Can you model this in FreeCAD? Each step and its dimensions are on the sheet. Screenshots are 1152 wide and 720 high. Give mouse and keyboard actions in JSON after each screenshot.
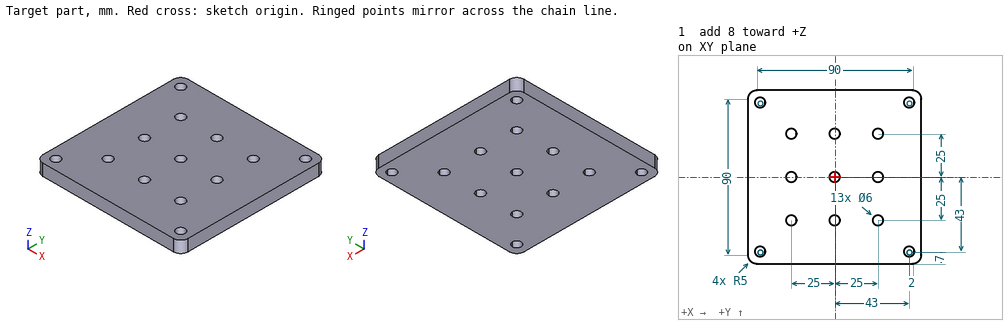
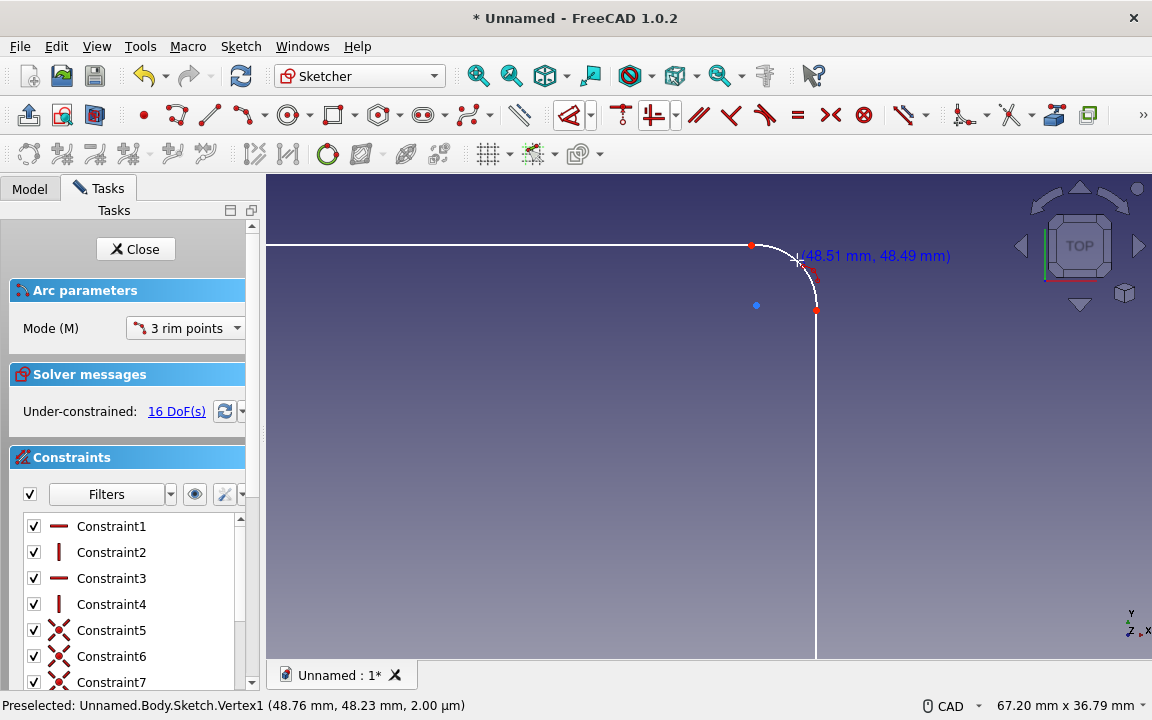
{"action": "left_click", "coordinate": [288, 116]}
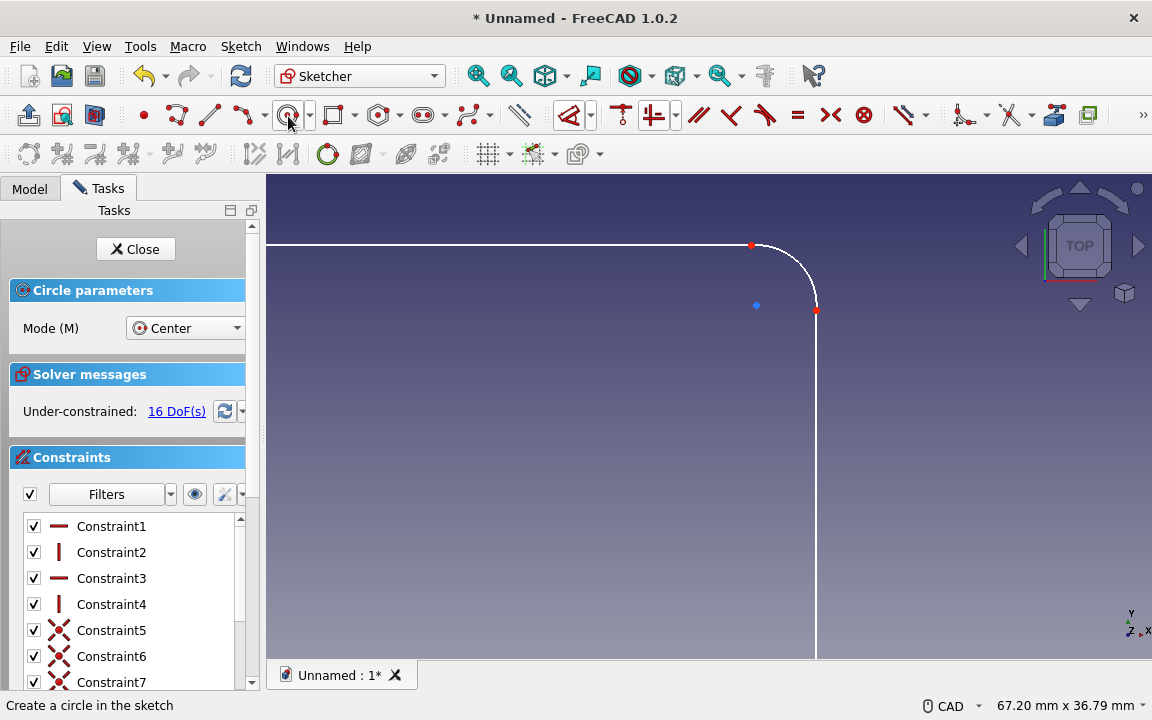
{"action": "scroll", "coordinate": [799, 258], "scroll_direction": "down", "scroll_amount": 7}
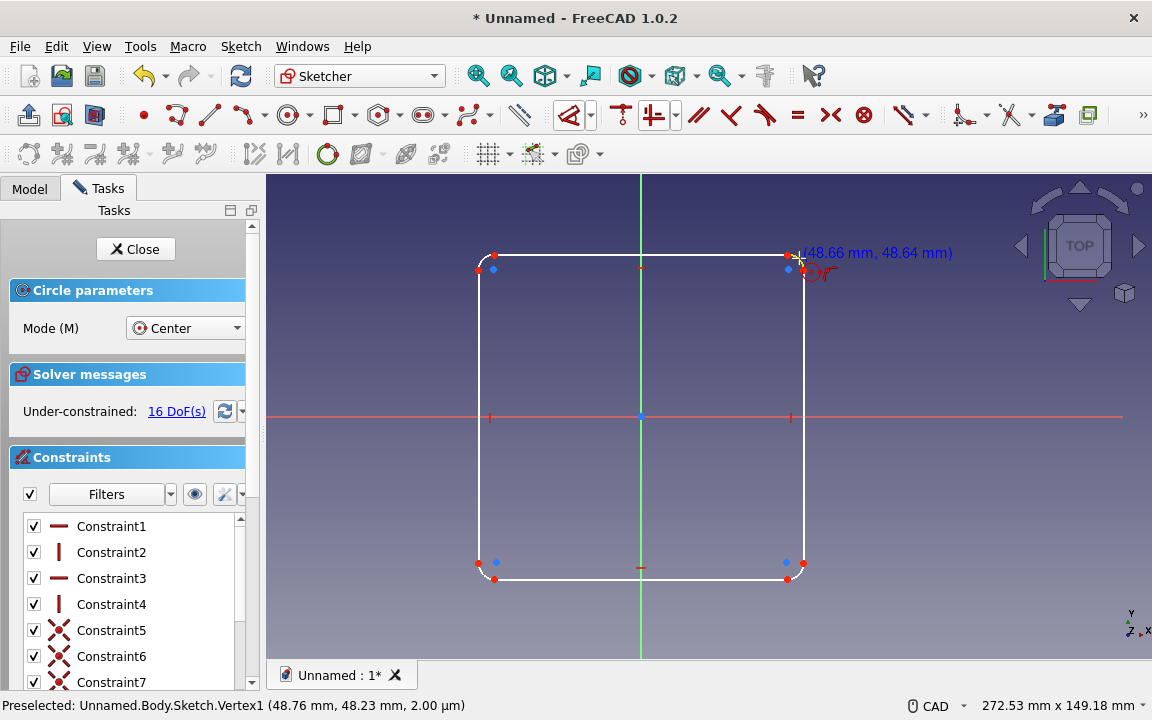
{"action": "scroll", "coordinate": [781, 556], "scroll_direction": "up", "scroll_amount": 5}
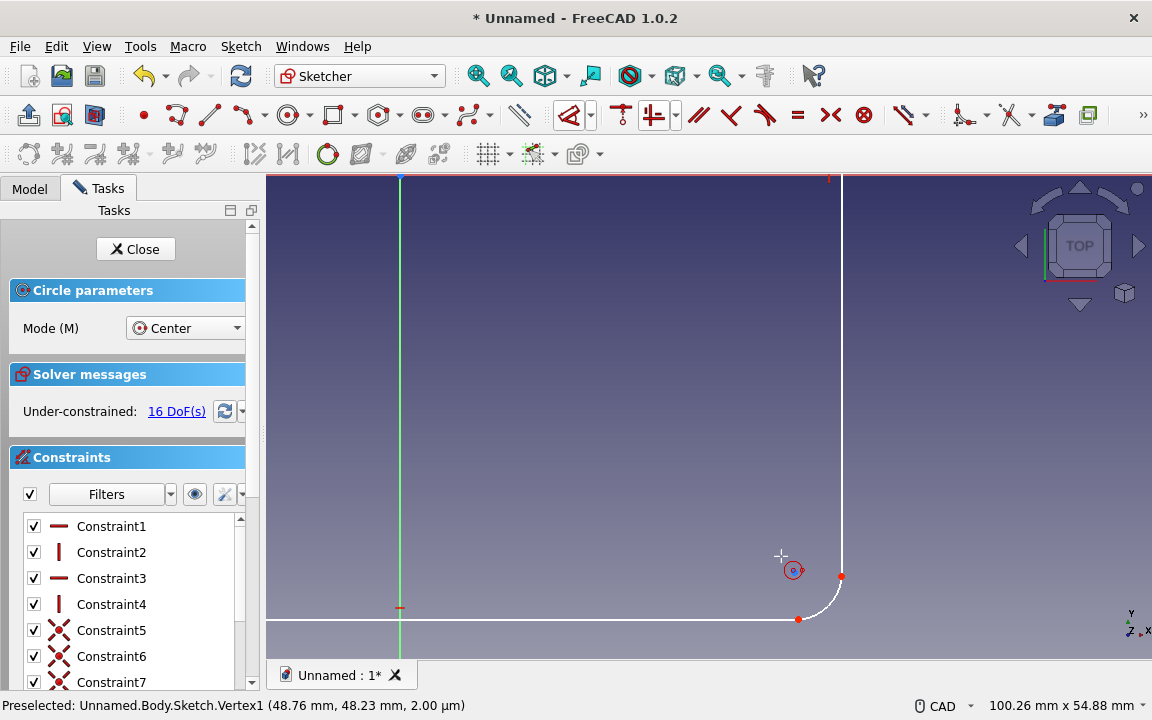
{"action": "left_click", "coordinate": [780, 555]}
{"action": "left_click", "coordinate": [799, 537]}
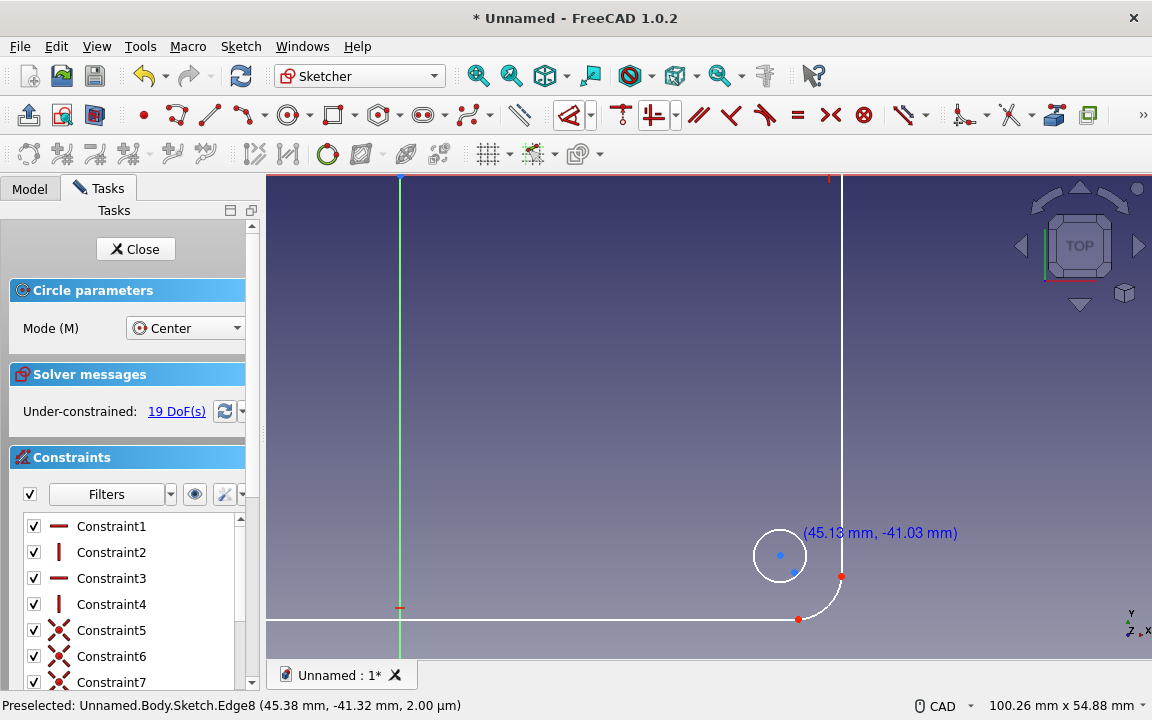
{"action": "left_click", "coordinate": [621, 396]}
{"action": "left_click", "coordinate": [640, 378]}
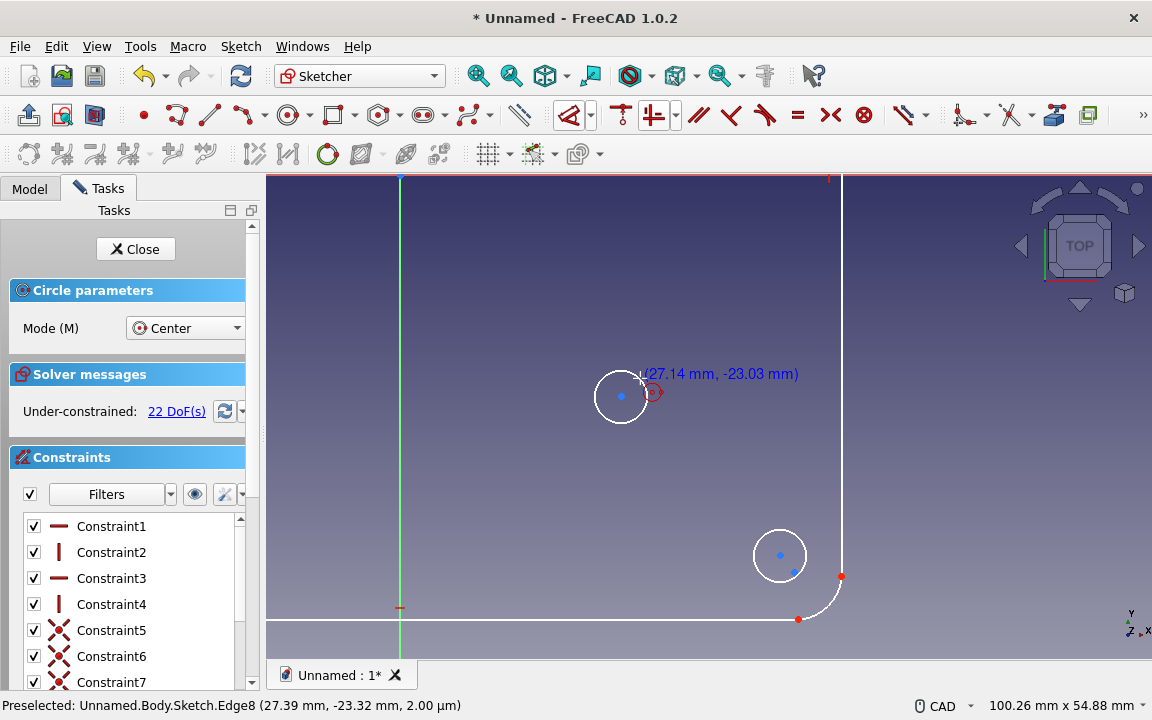
{"action": "left_click", "coordinate": [400, 396]}
{"action": "left_click", "coordinate": [419, 378]}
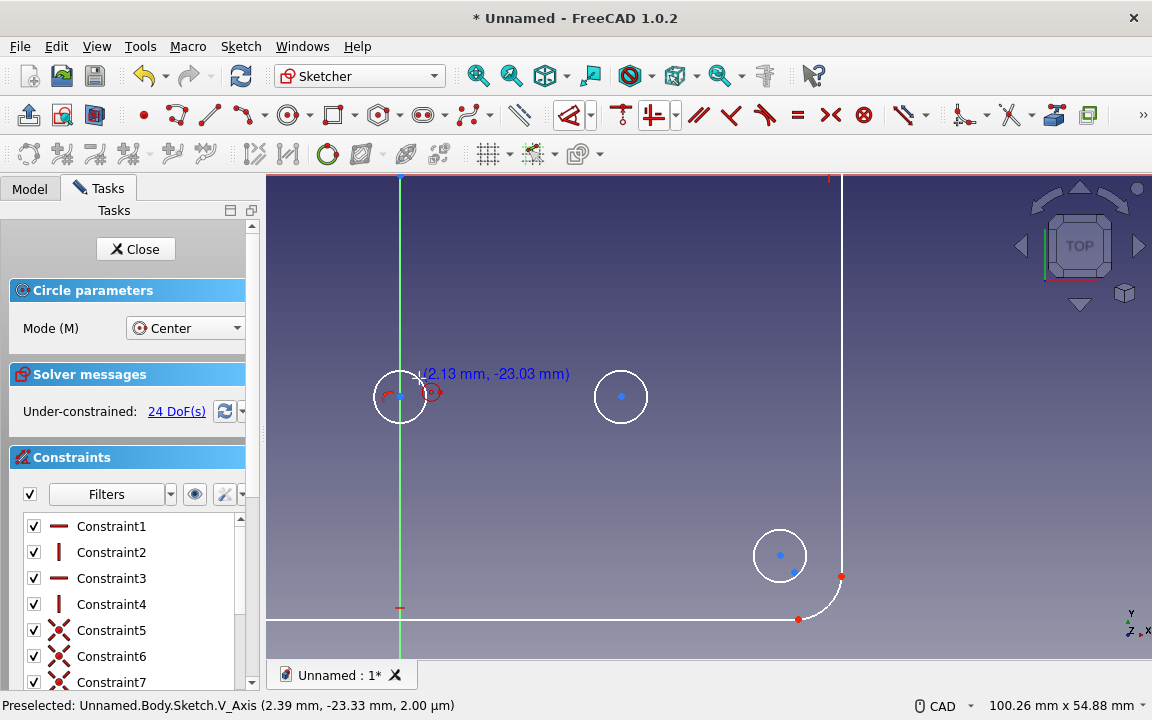
{"action": "scroll", "coordinate": [780, 557], "scroll_direction": "down", "scroll_amount": 5}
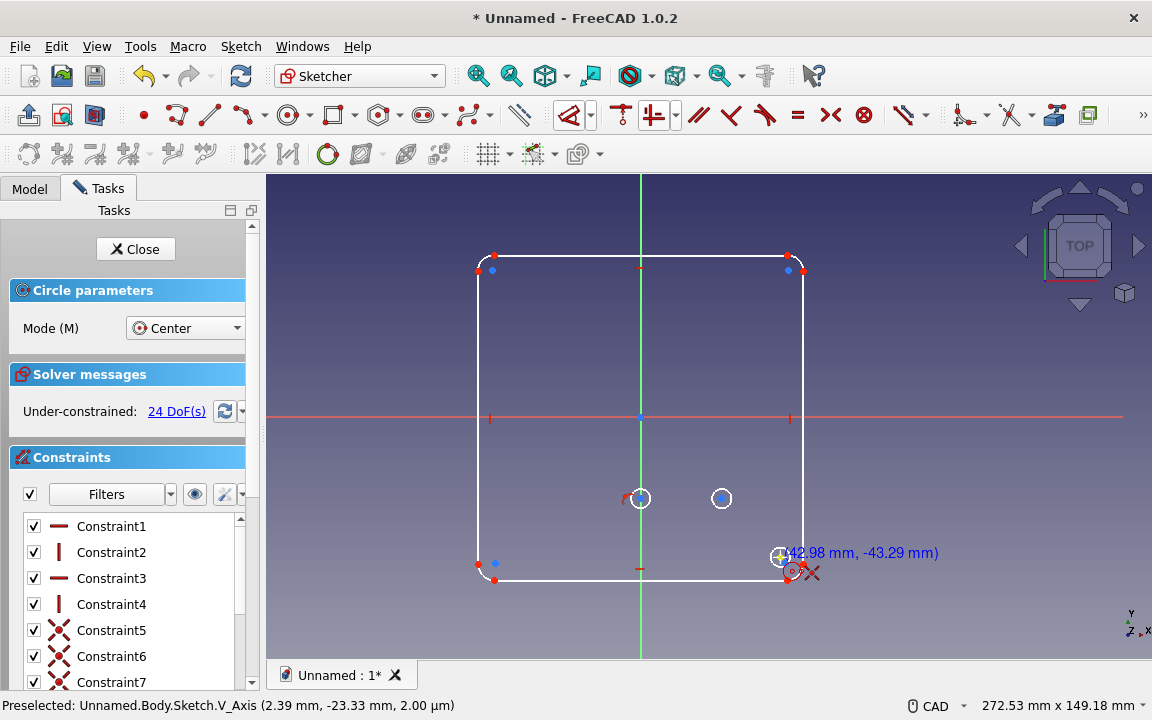
{"action": "scroll", "coordinate": [501, 557], "scroll_direction": "up", "scroll_amount": 5}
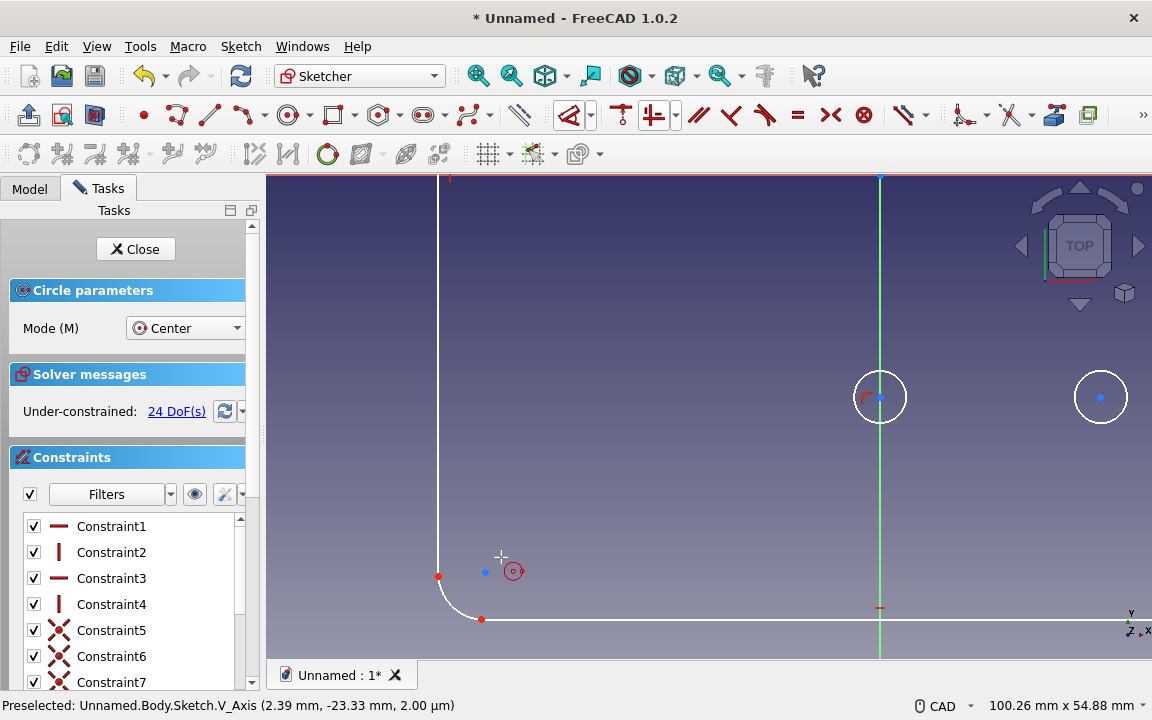
{"action": "left_click", "coordinate": [500, 555]}
{"action": "left_click", "coordinate": [519, 537]}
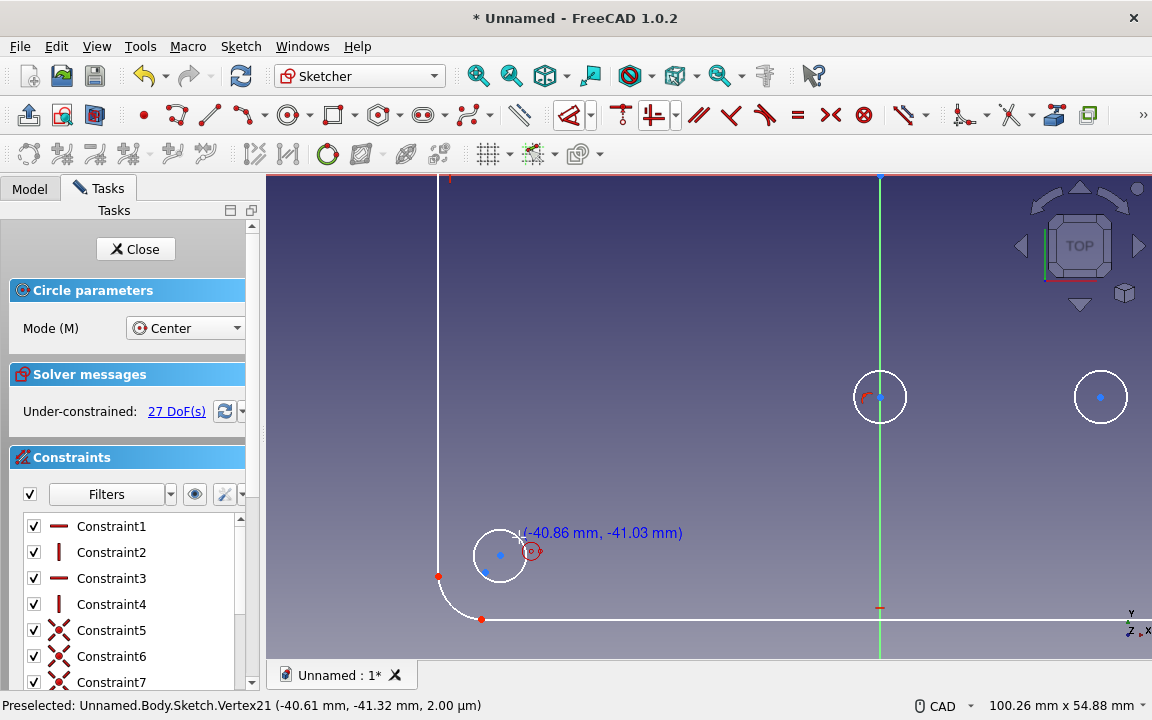
{"action": "left_click", "coordinate": [659, 396]}
{"action": "left_click", "coordinate": [678, 378]}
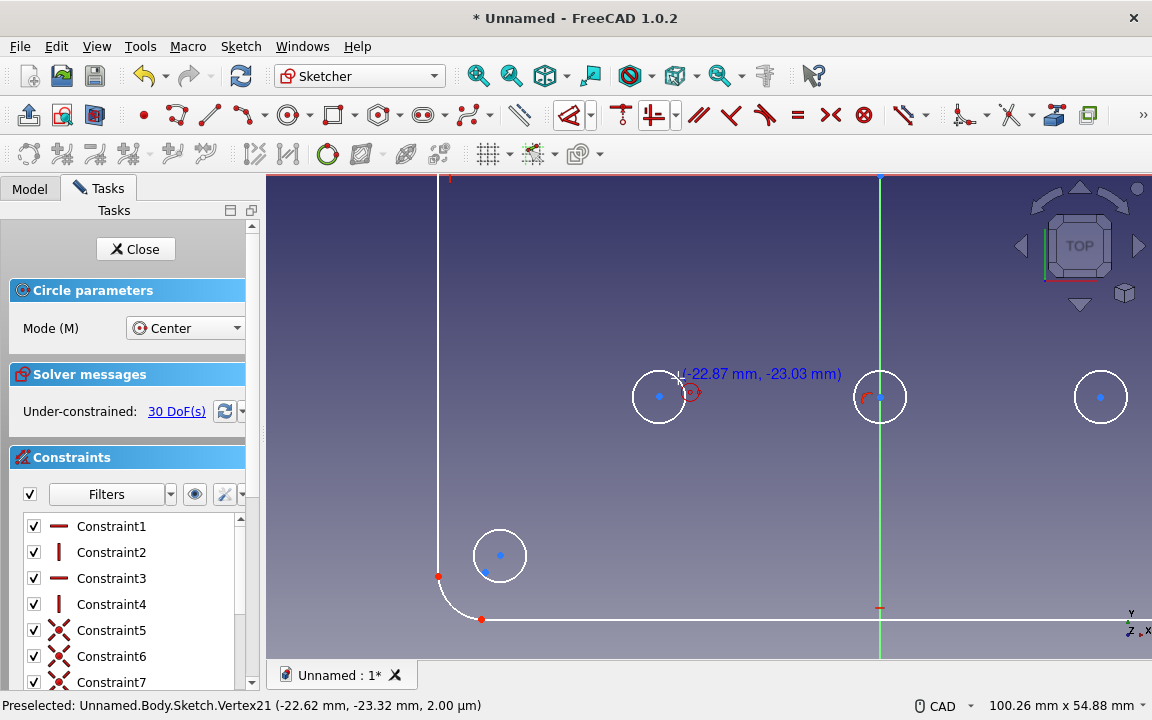
{"action": "scroll", "coordinate": [501, 557], "scroll_direction": "down", "scroll_amount": 5}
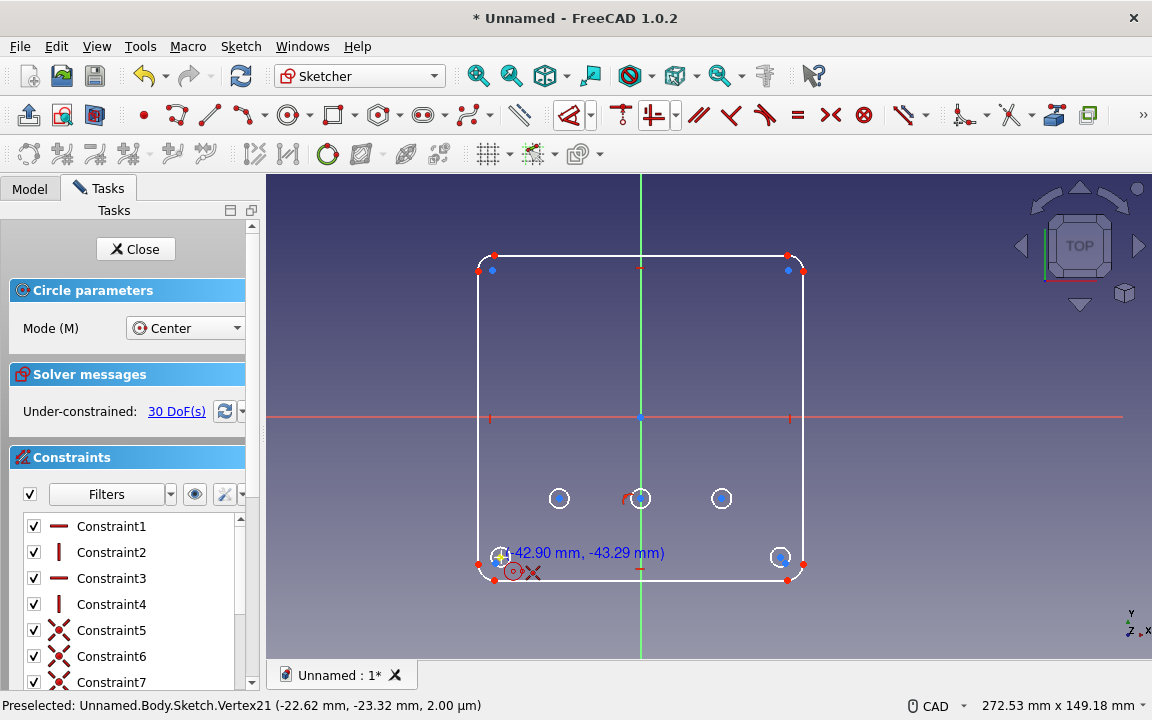
{"action": "scroll", "coordinate": [722, 417], "scroll_direction": "up", "scroll_amount": 5}